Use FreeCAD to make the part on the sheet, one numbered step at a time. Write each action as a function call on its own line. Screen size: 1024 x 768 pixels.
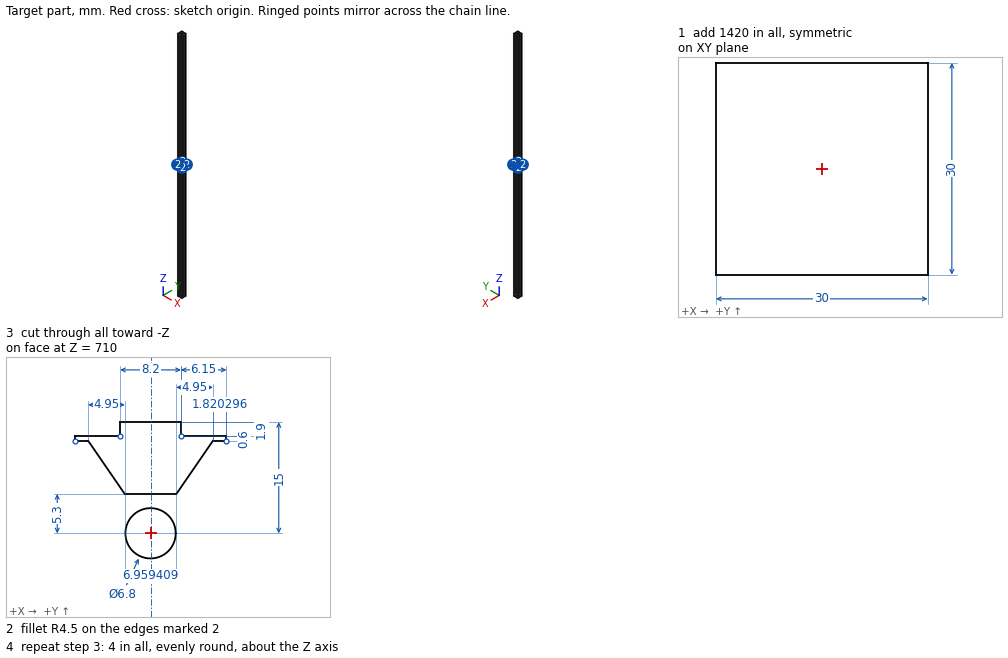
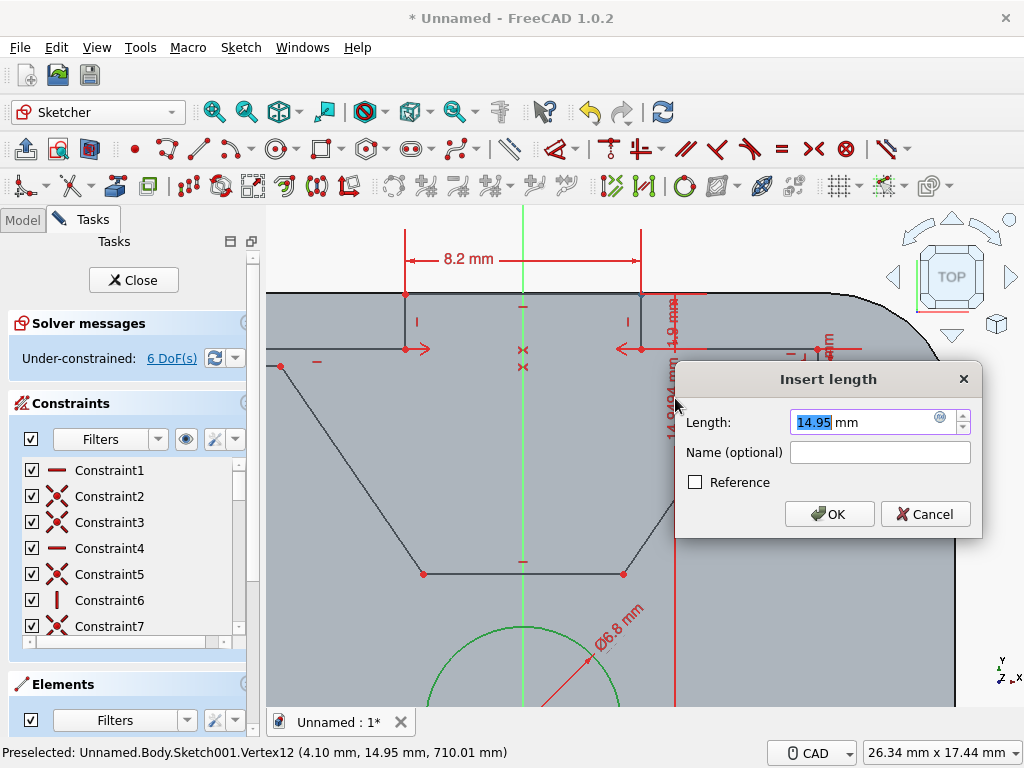
text(15)
key(Return)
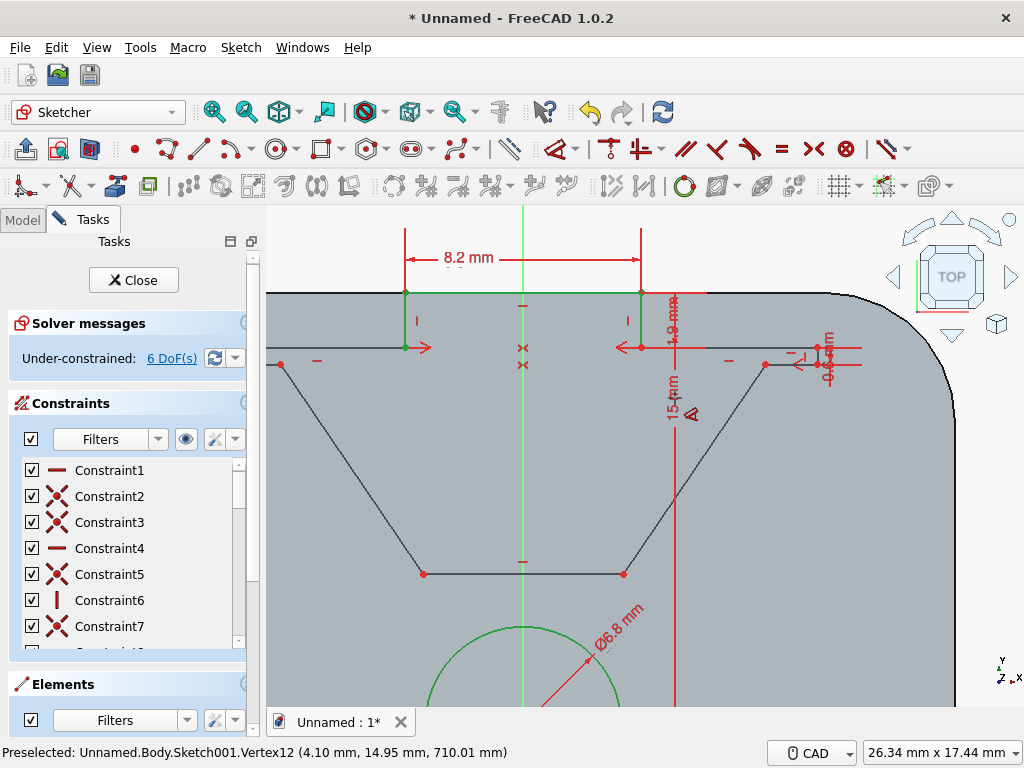
click(765, 348)
click(770, 314)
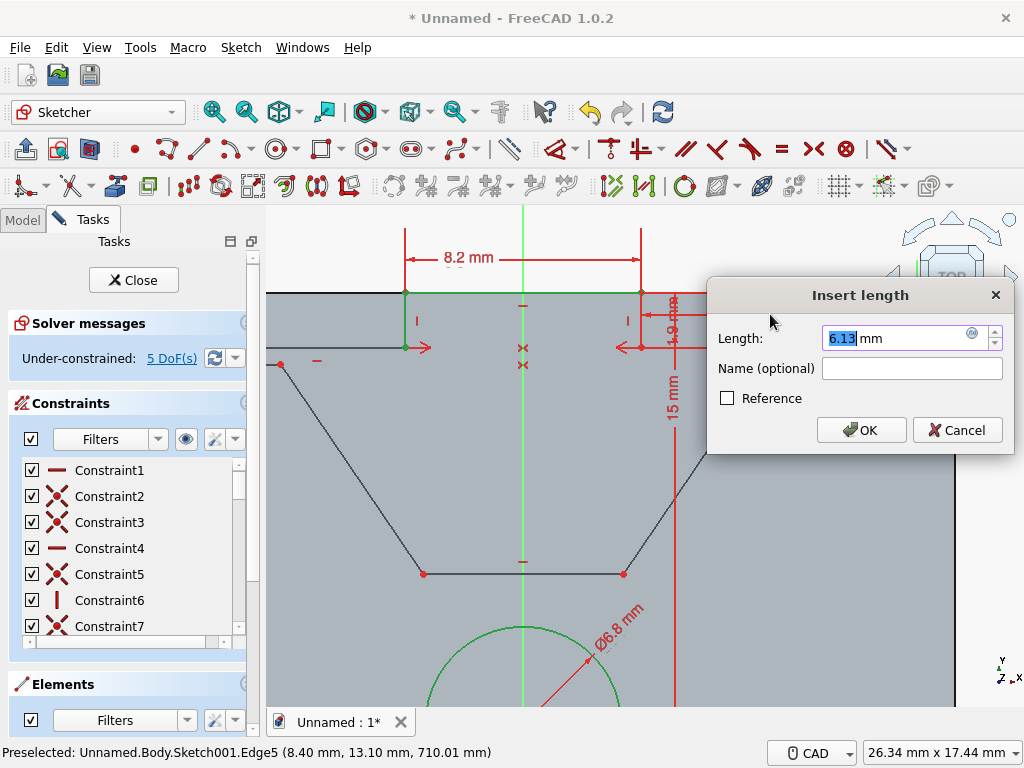
text(6.15)
key(Return)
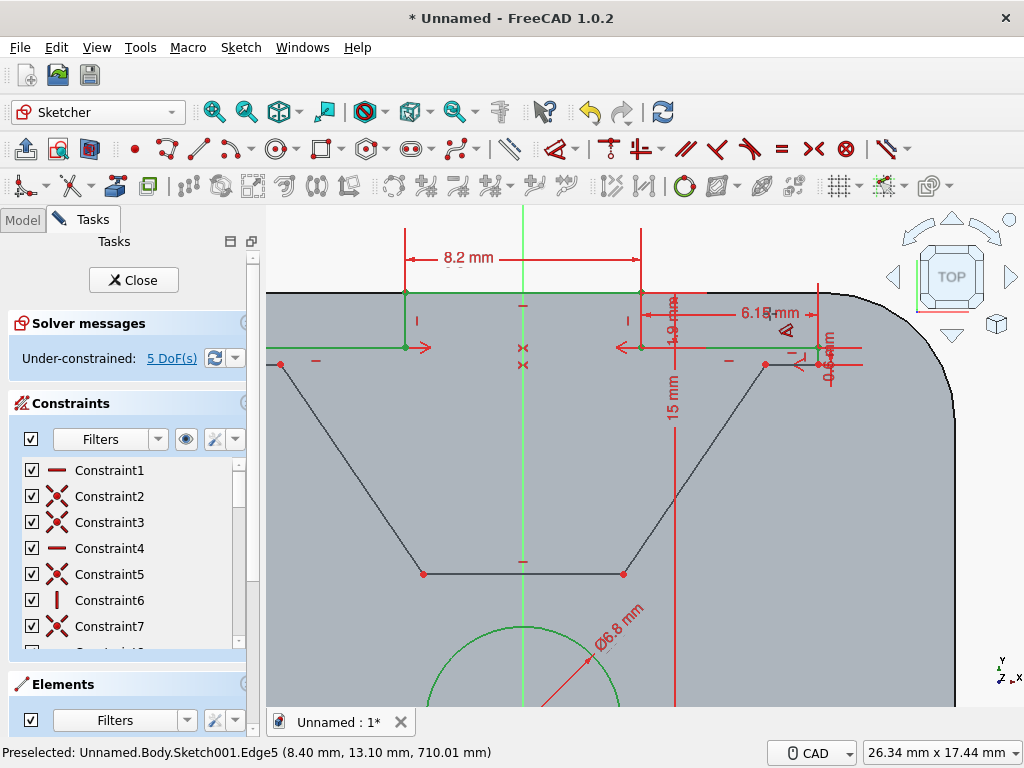
click(423, 574)
click(389, 627)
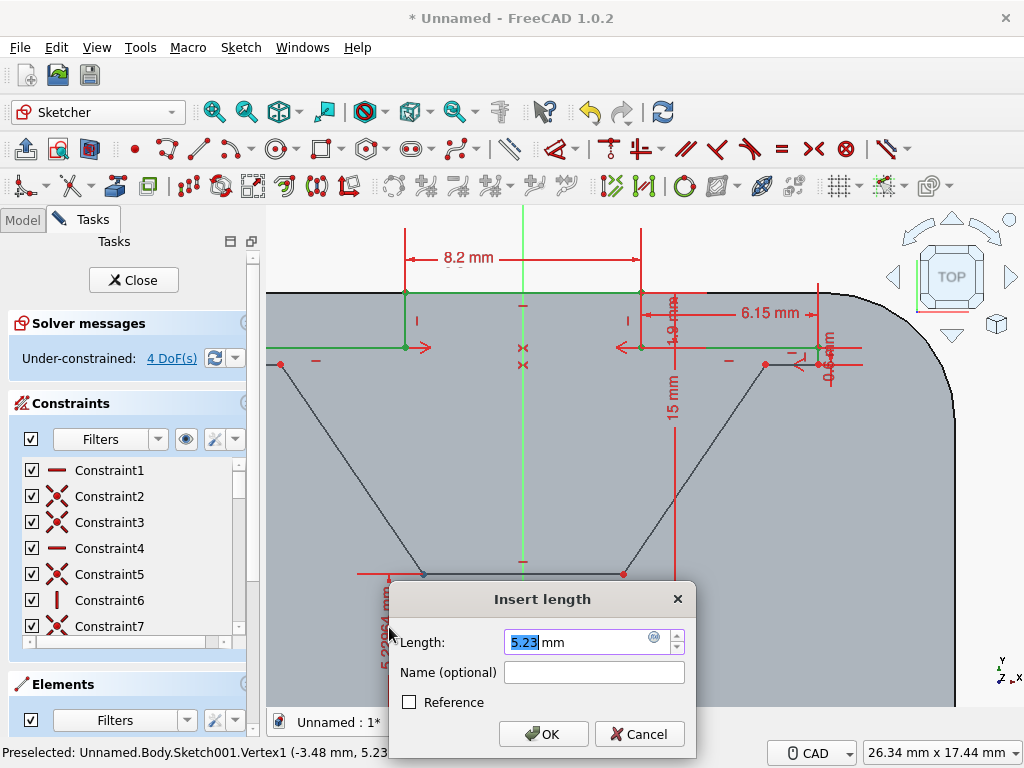
text(5.3)
key(Return)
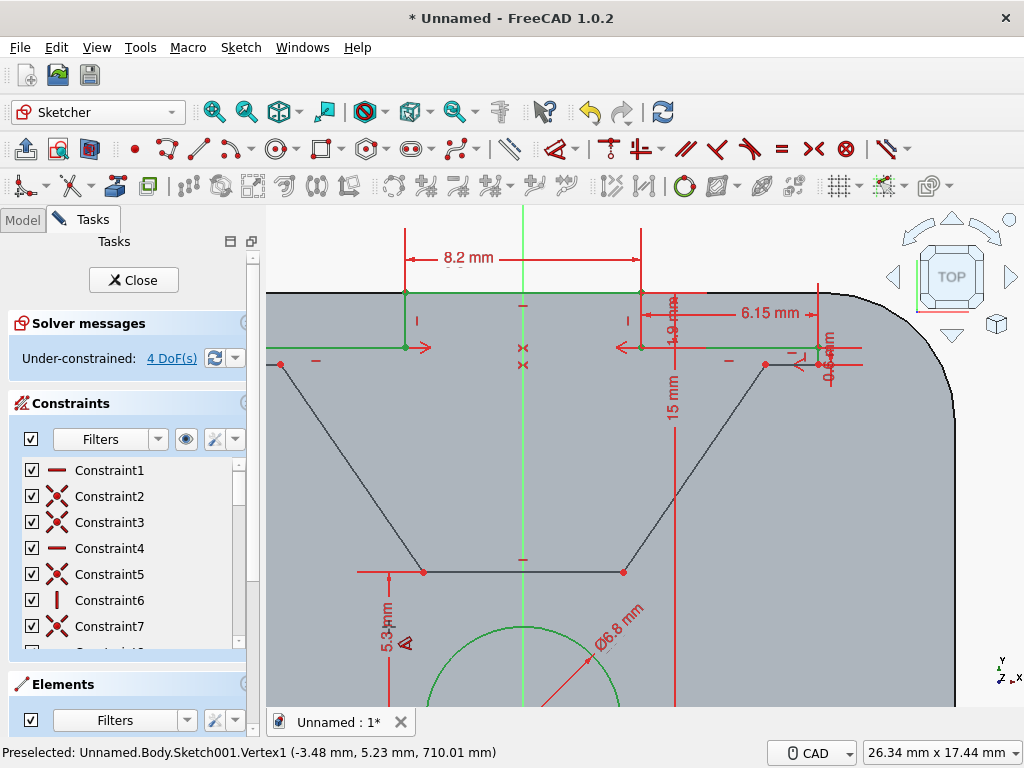
click(666, 510)
click(695, 606)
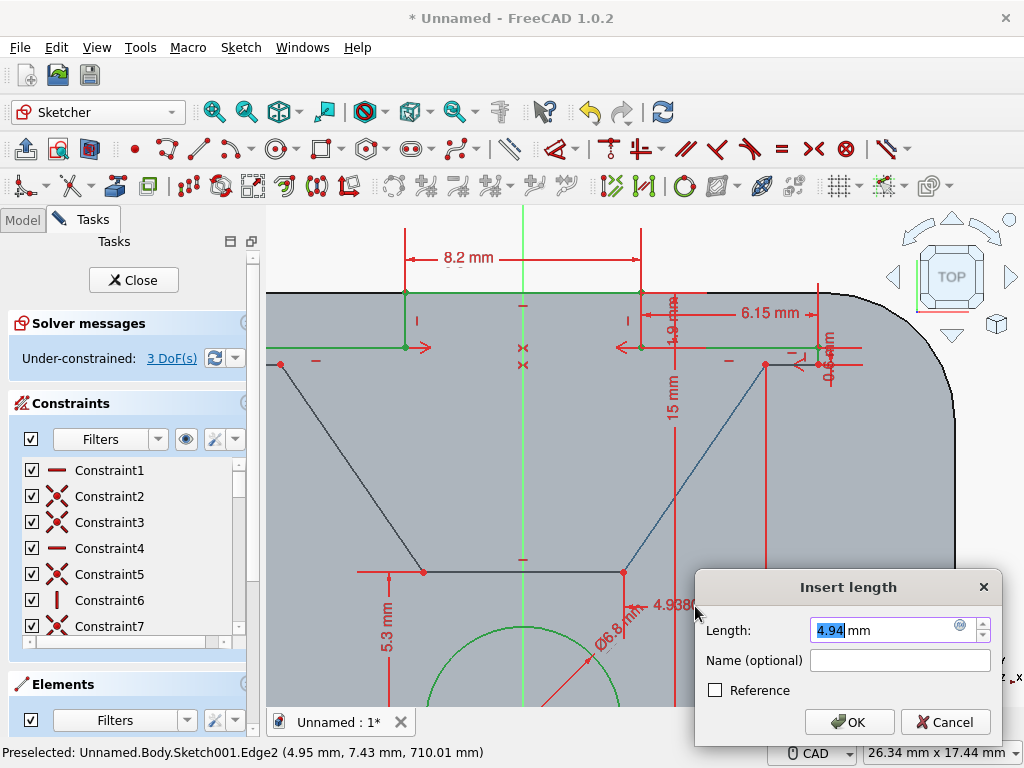
text(4.95)
key(Return)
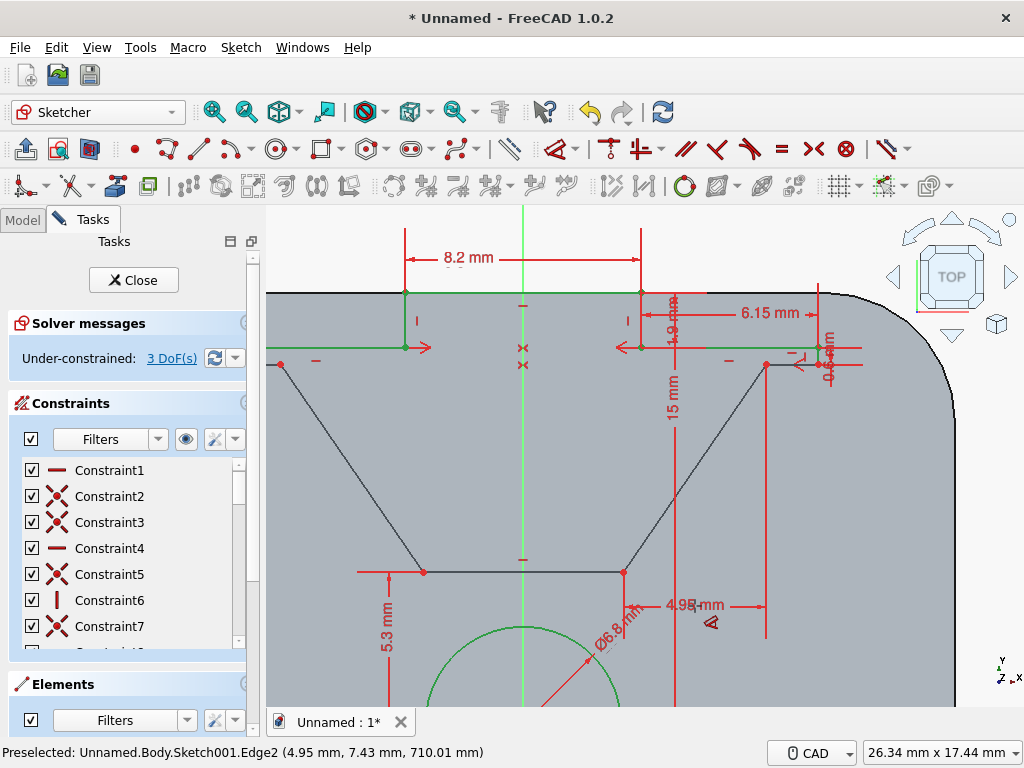
click(324, 427)
click(359, 331)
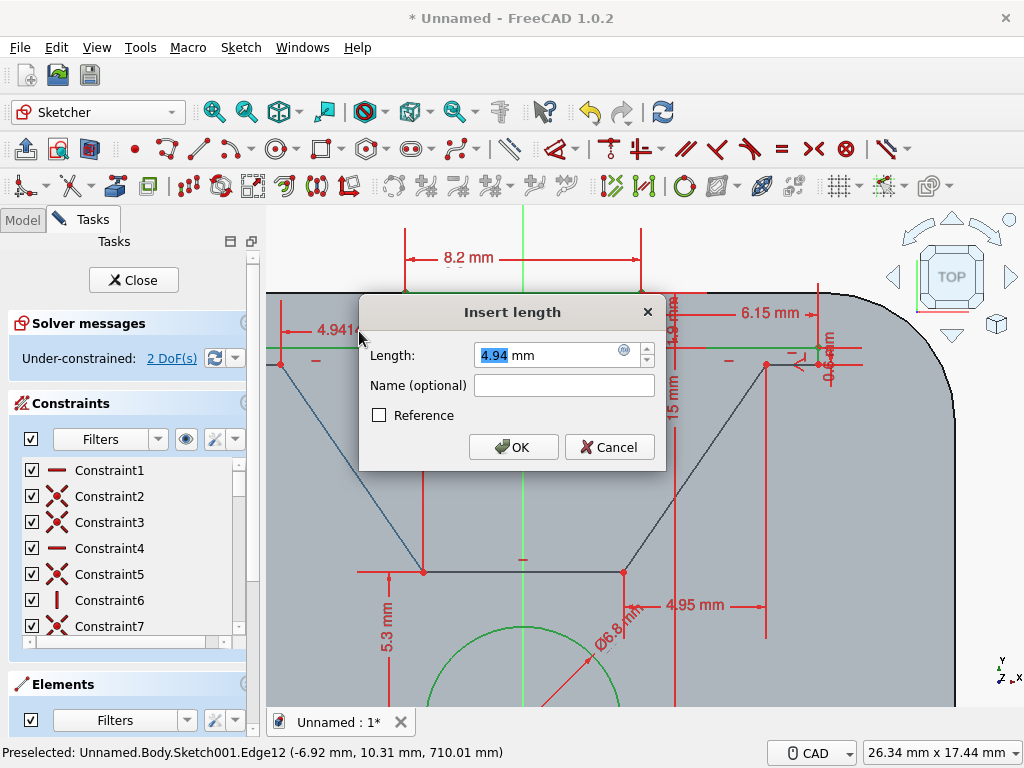
text(4.95)
key(Return)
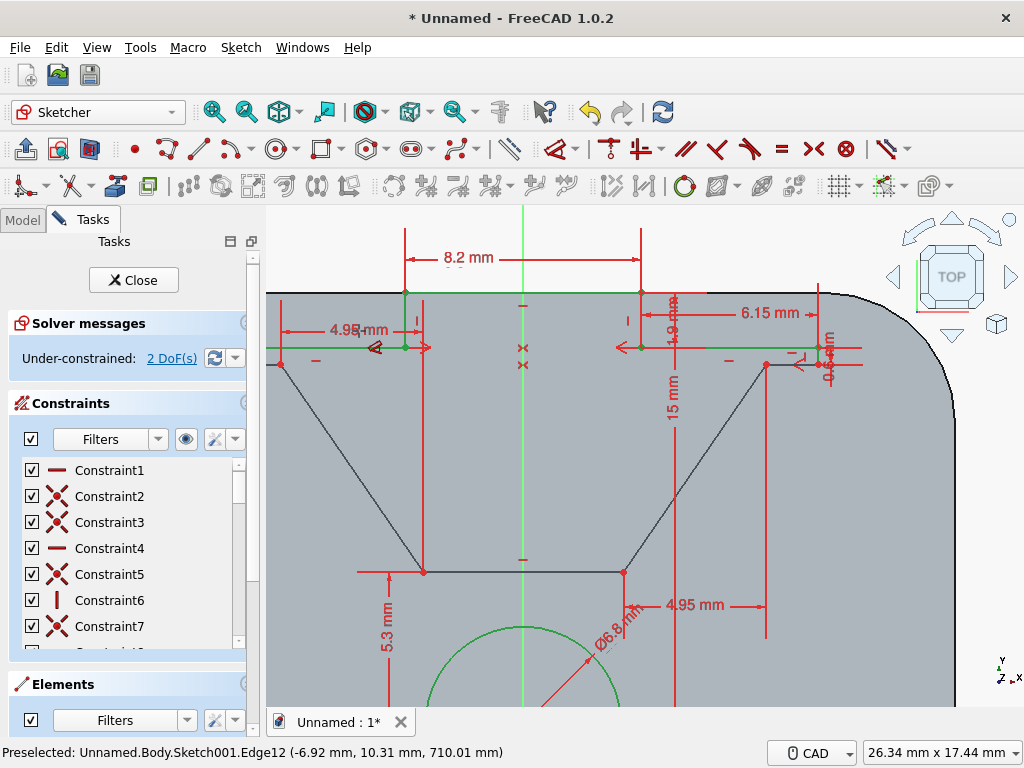
click(483, 572)
click(477, 606)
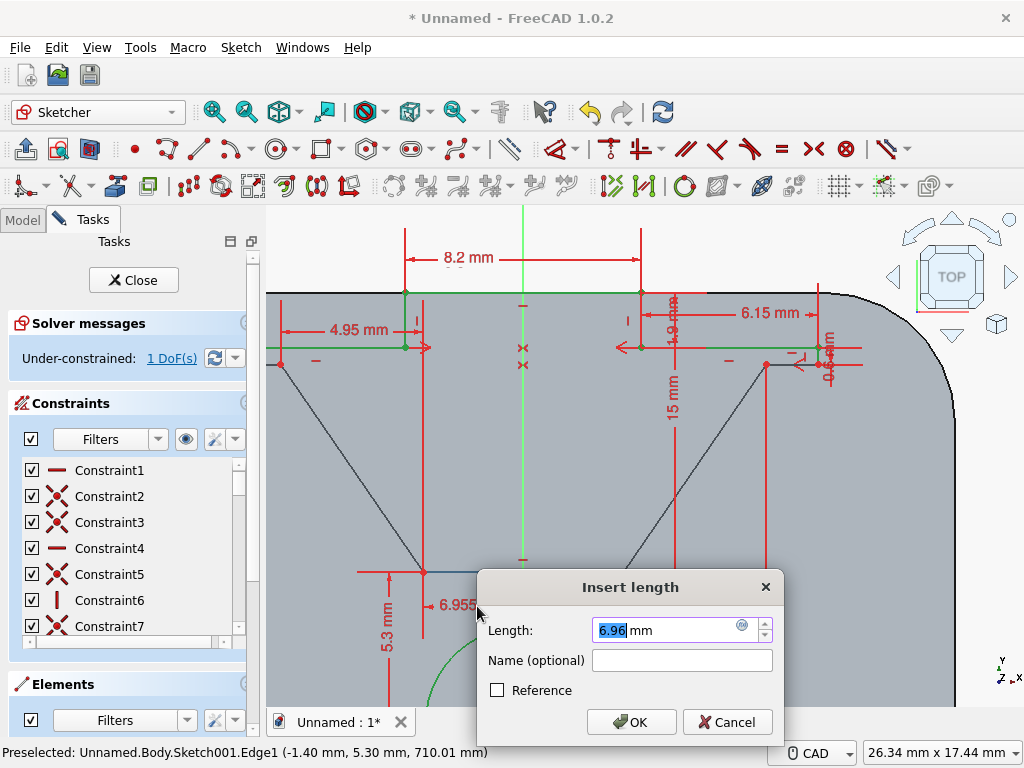
text(6.959409)
key(Return)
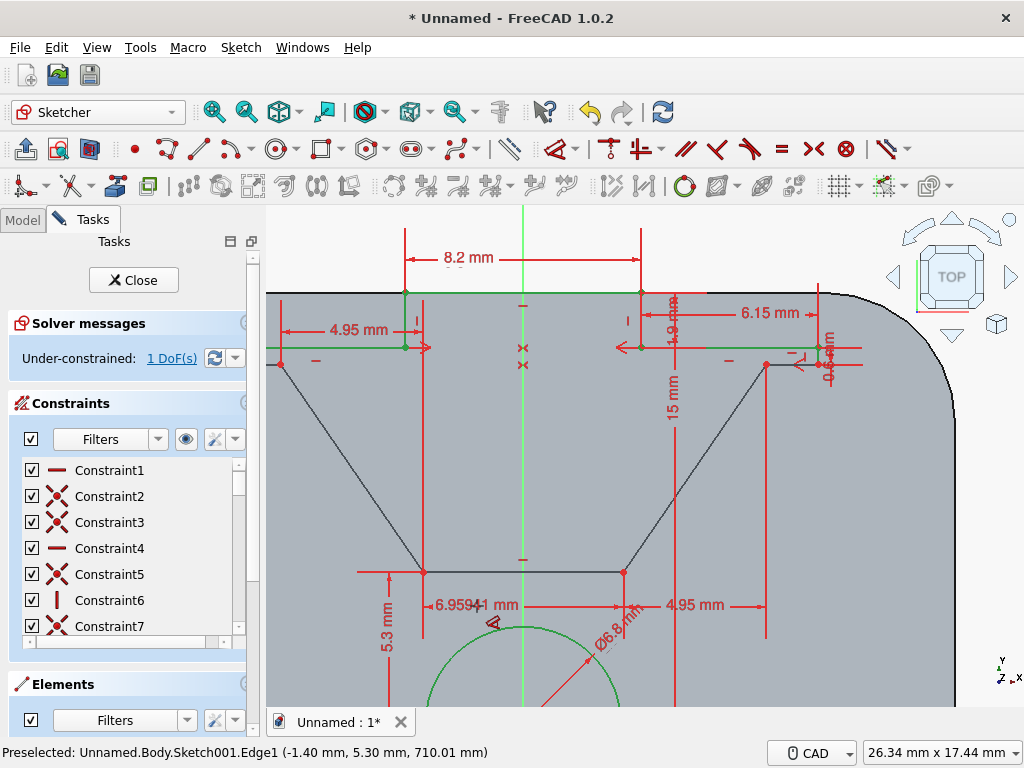
click(782, 365)
click(792, 399)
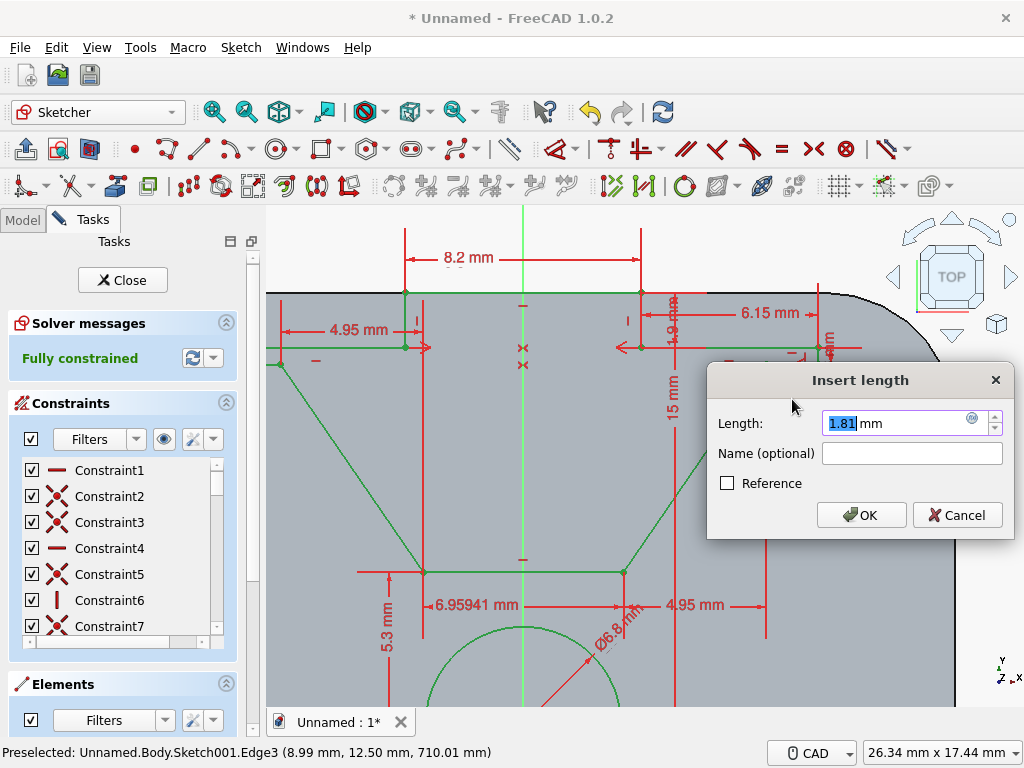
text(1.820296)
key(Return)
key(Escape)